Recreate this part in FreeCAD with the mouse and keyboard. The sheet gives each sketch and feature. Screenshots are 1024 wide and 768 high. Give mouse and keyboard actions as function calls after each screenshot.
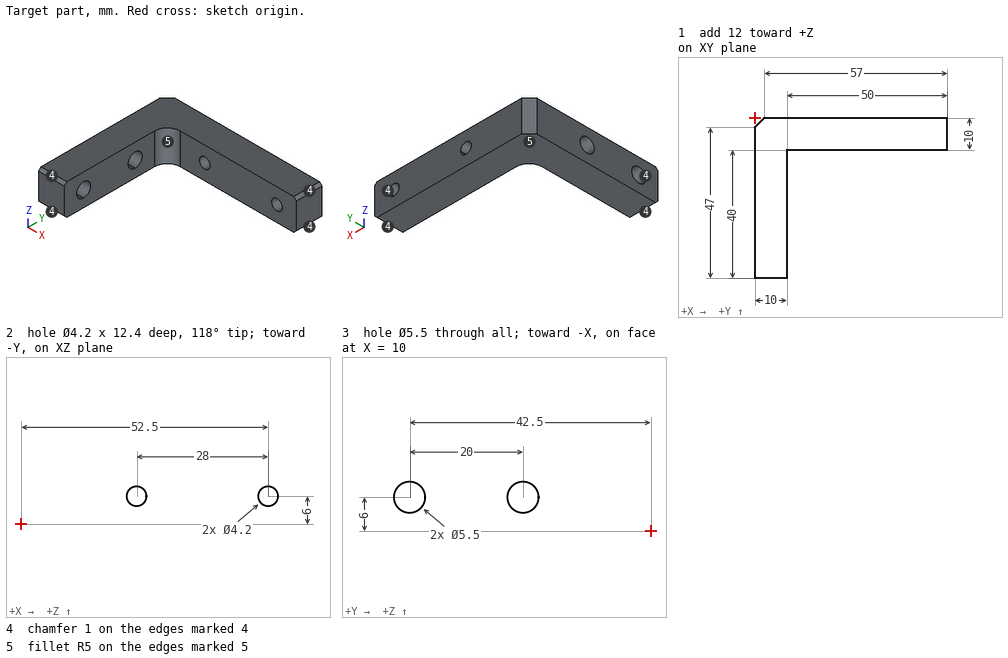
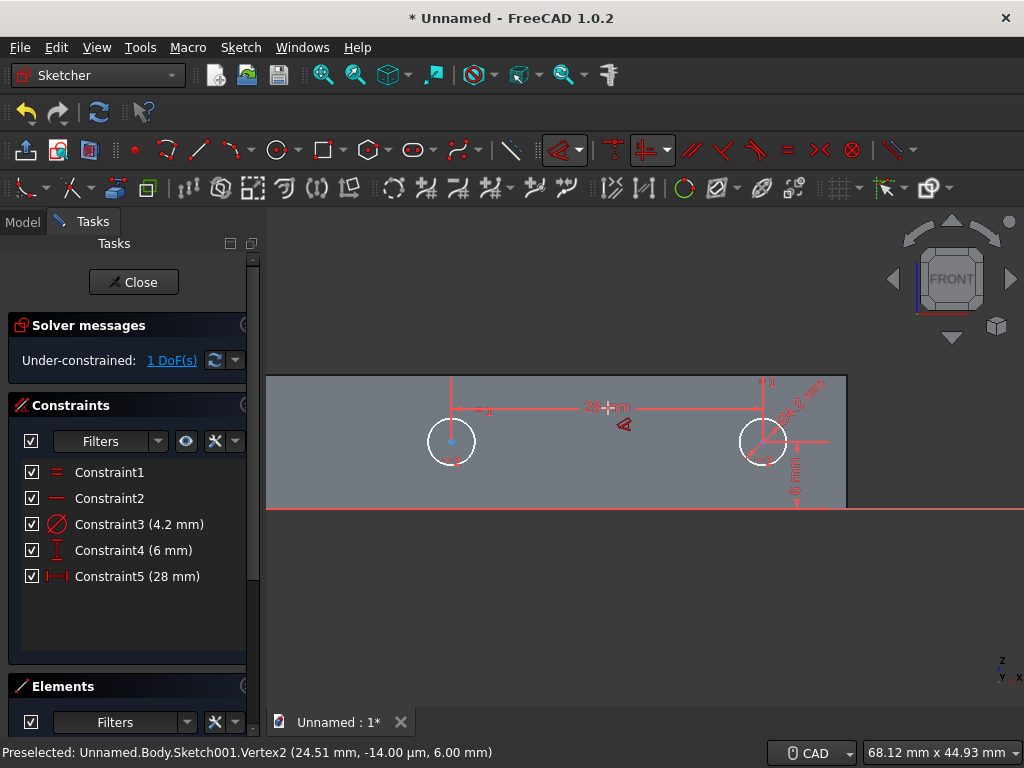
click(763, 442)
click(529, 543)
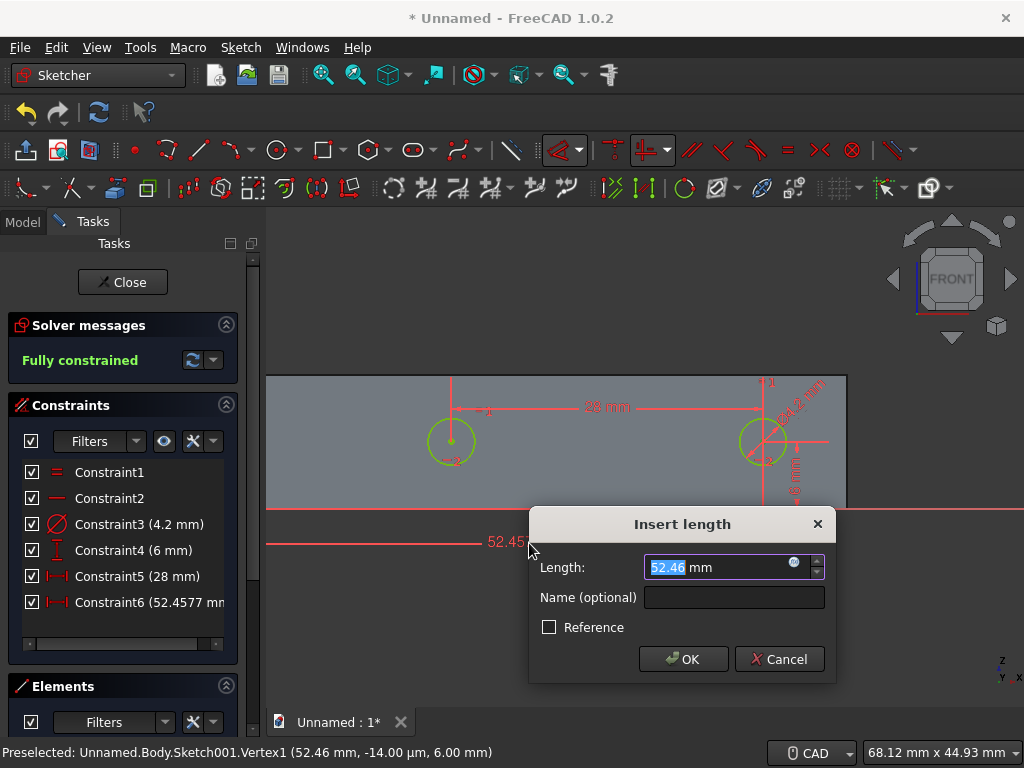
text(52.5)
key(Return)
key(Escape)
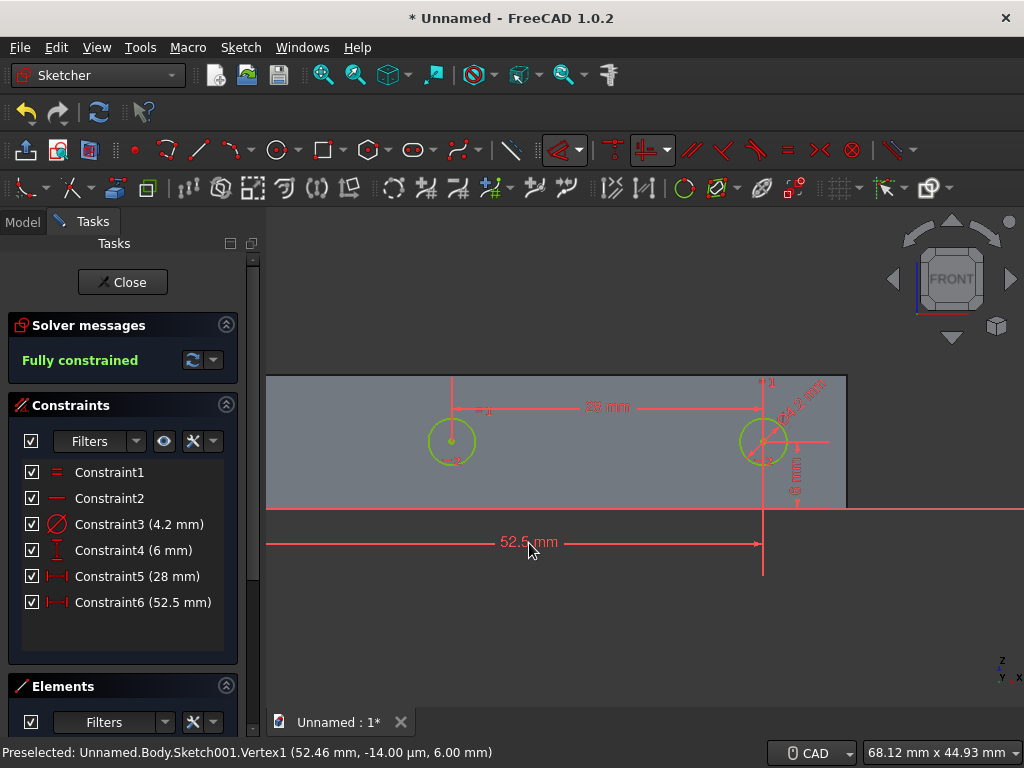
click(123, 282)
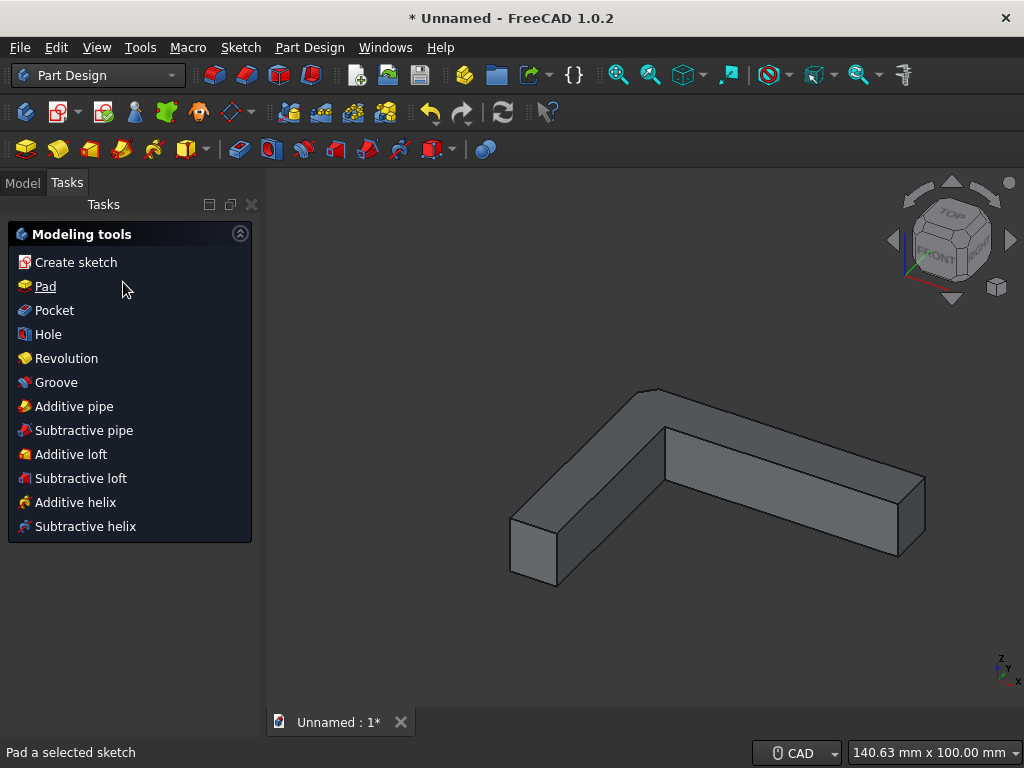
click(272, 150)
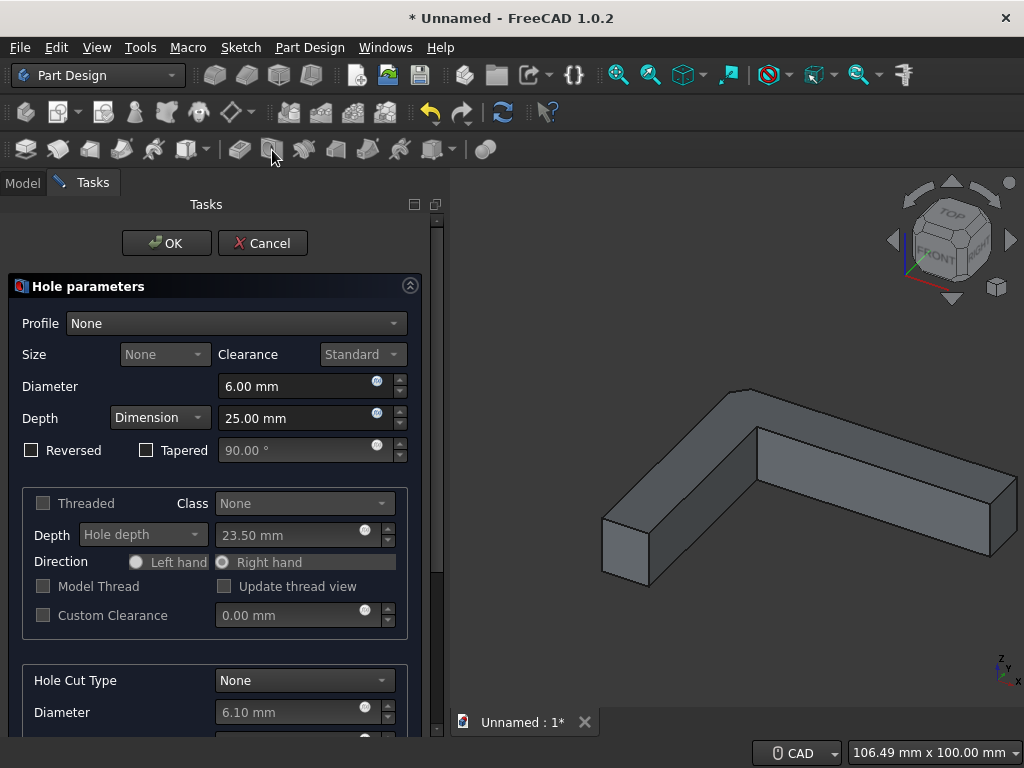
triple_click(305, 386)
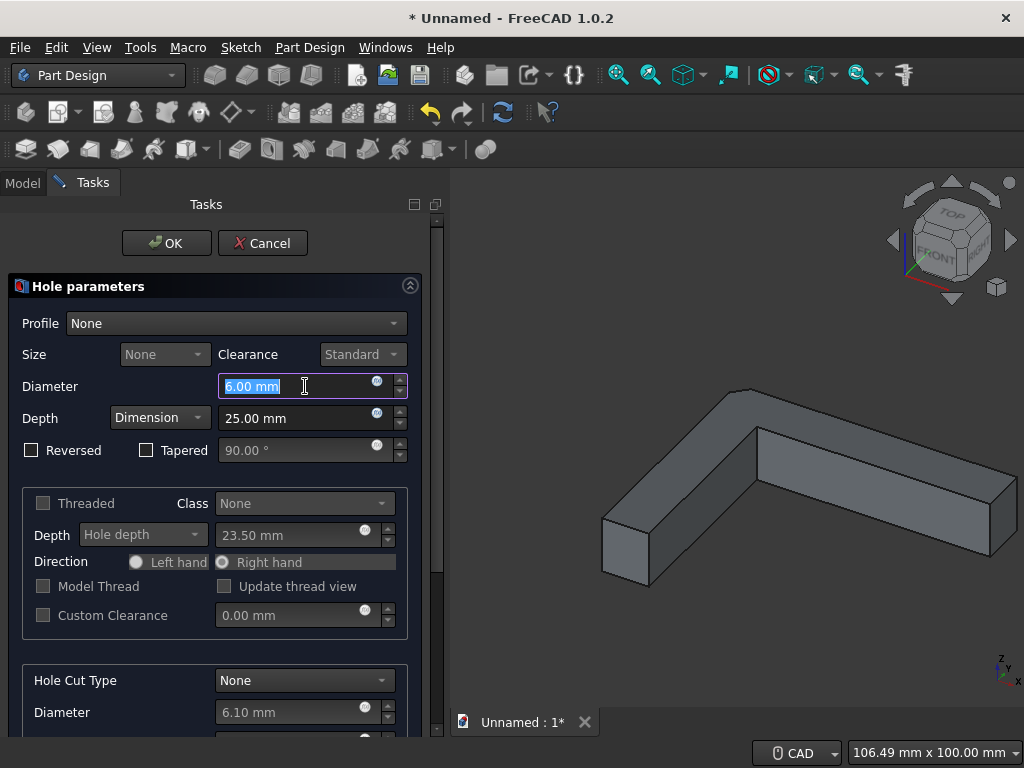
text(4.2)
key(Tab)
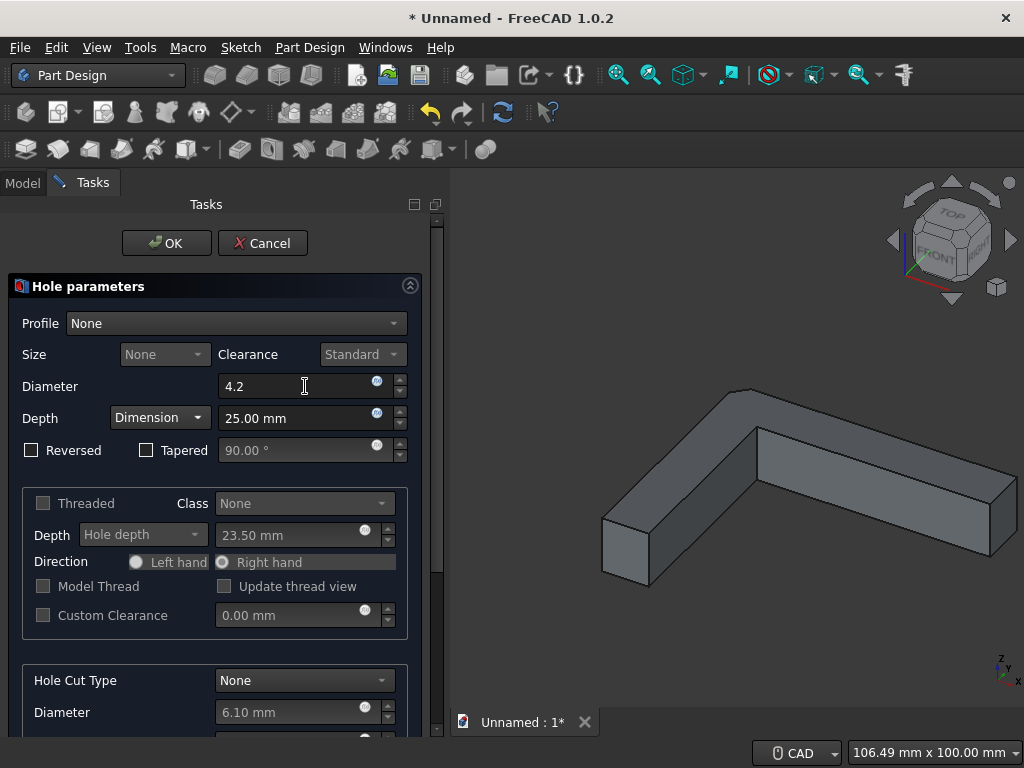
triple_click(305, 418)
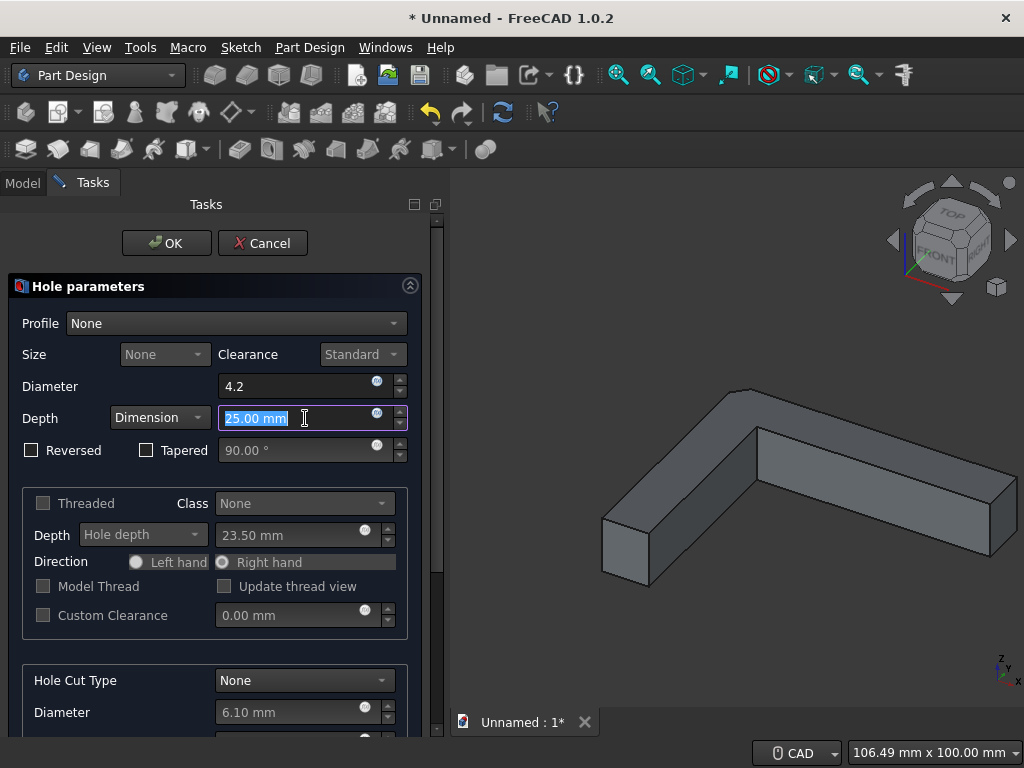
text(12.4)
key(Tab)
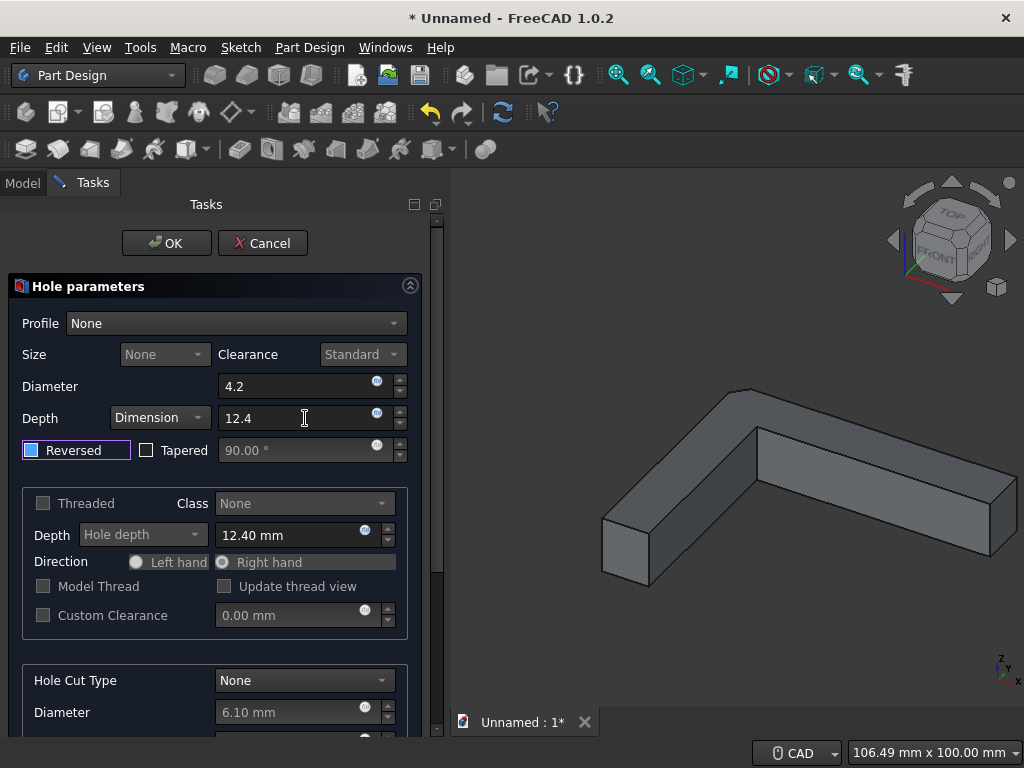
click(30, 450)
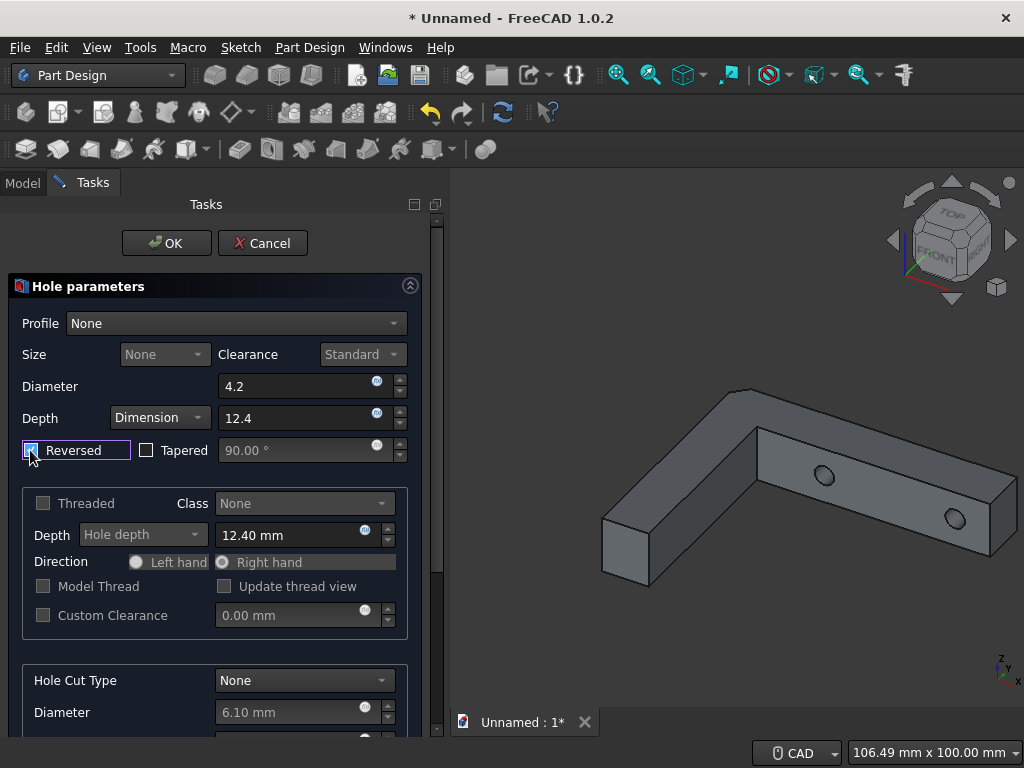
click(167, 243)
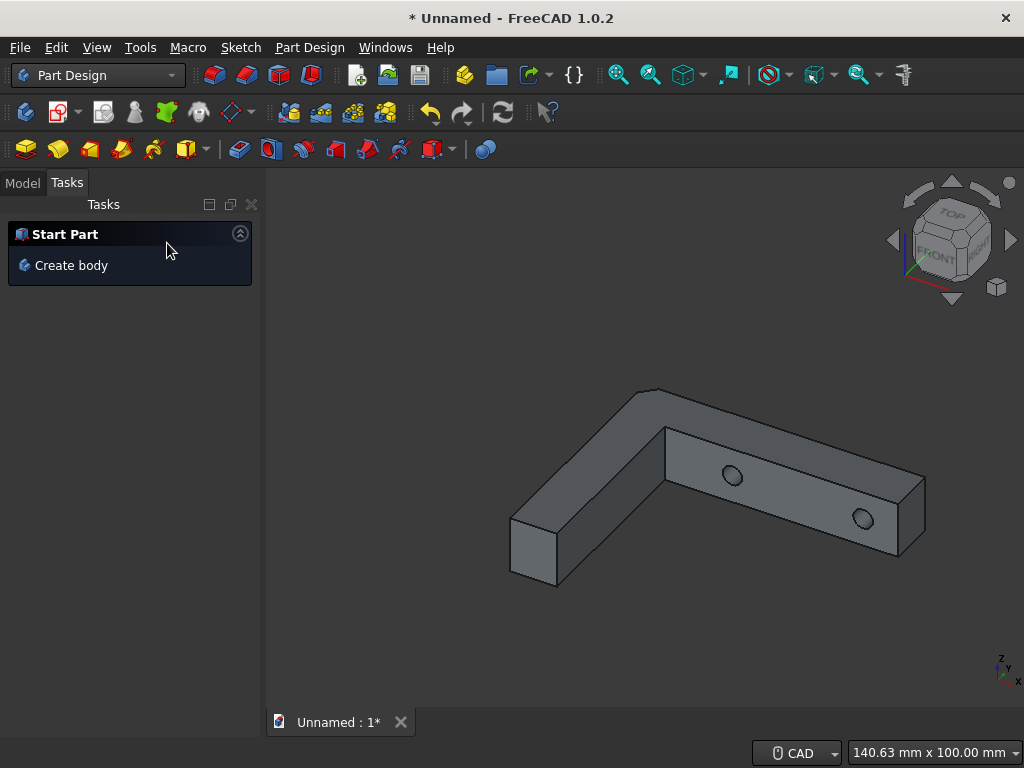
click(642, 475)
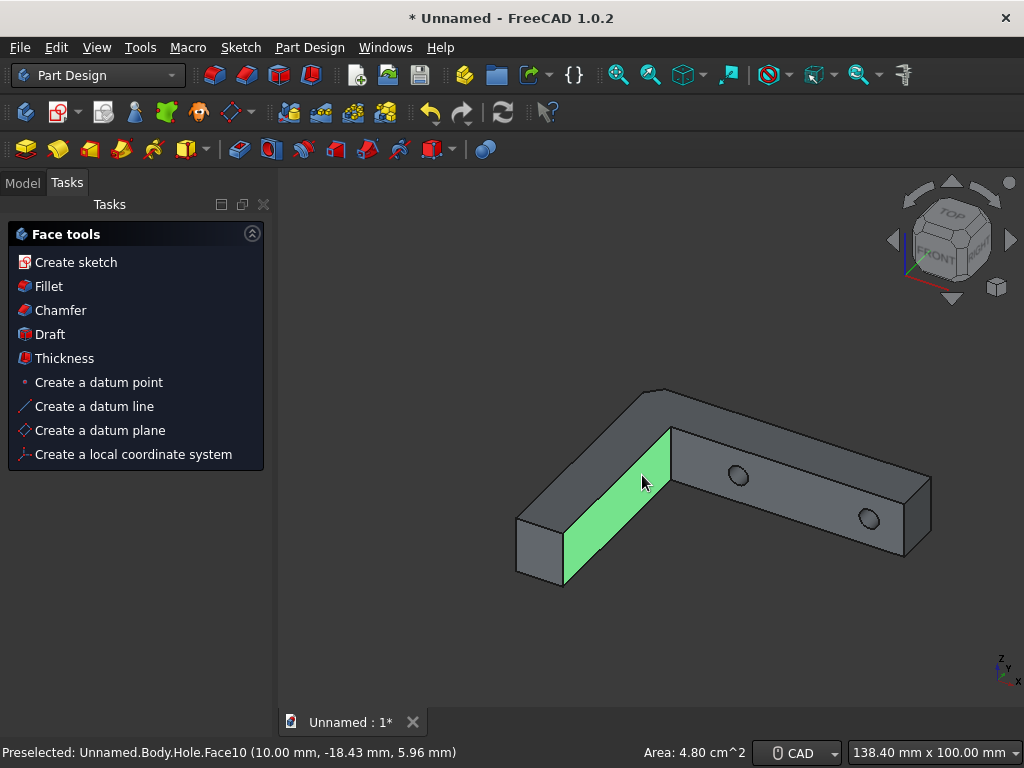
click(58, 112)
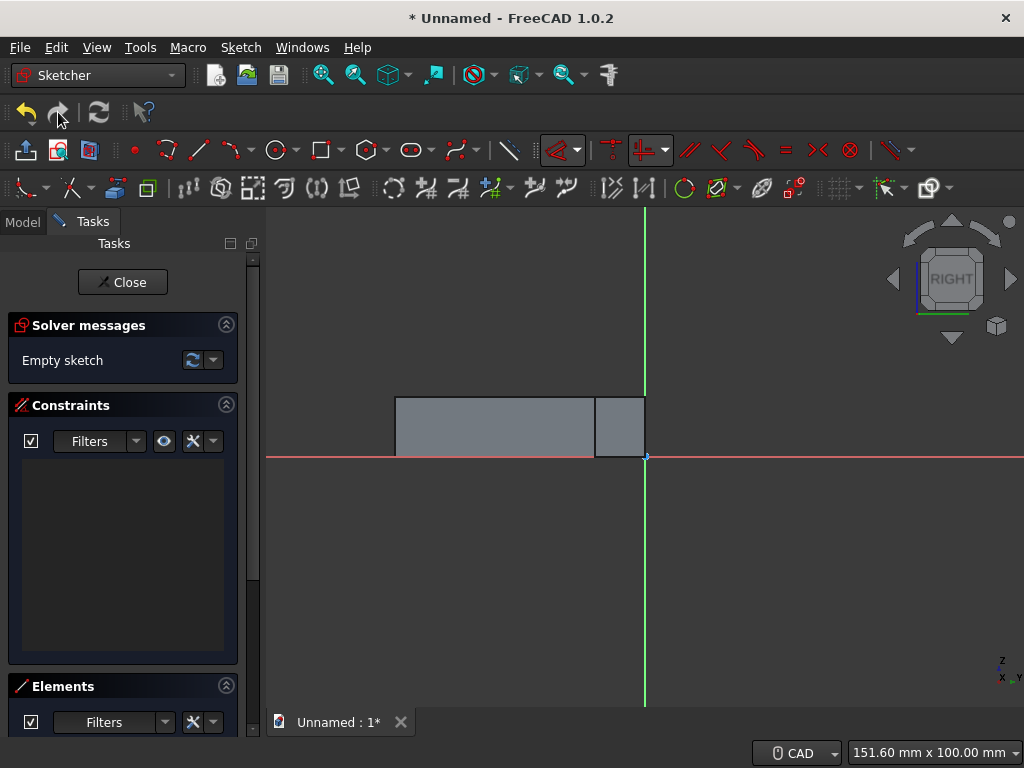
key(q)
key(s)